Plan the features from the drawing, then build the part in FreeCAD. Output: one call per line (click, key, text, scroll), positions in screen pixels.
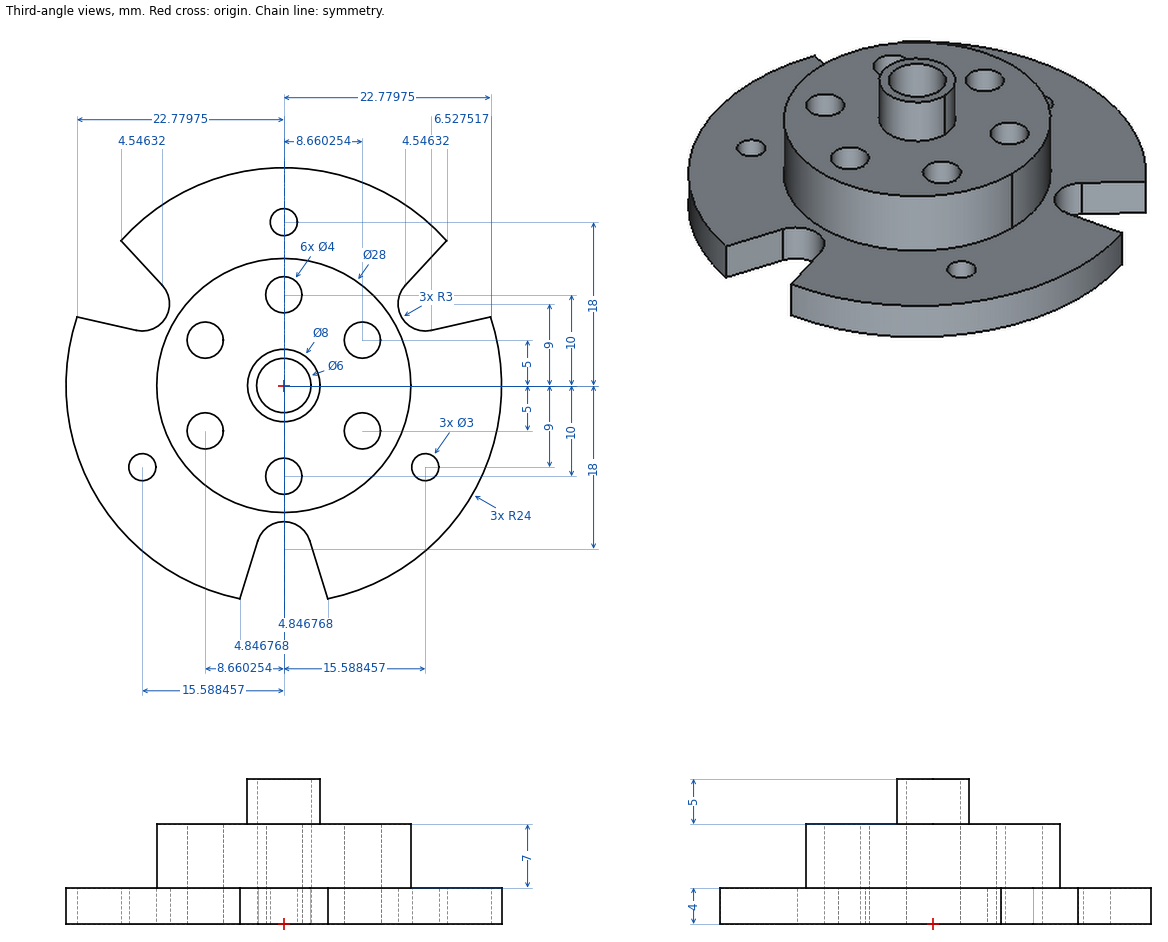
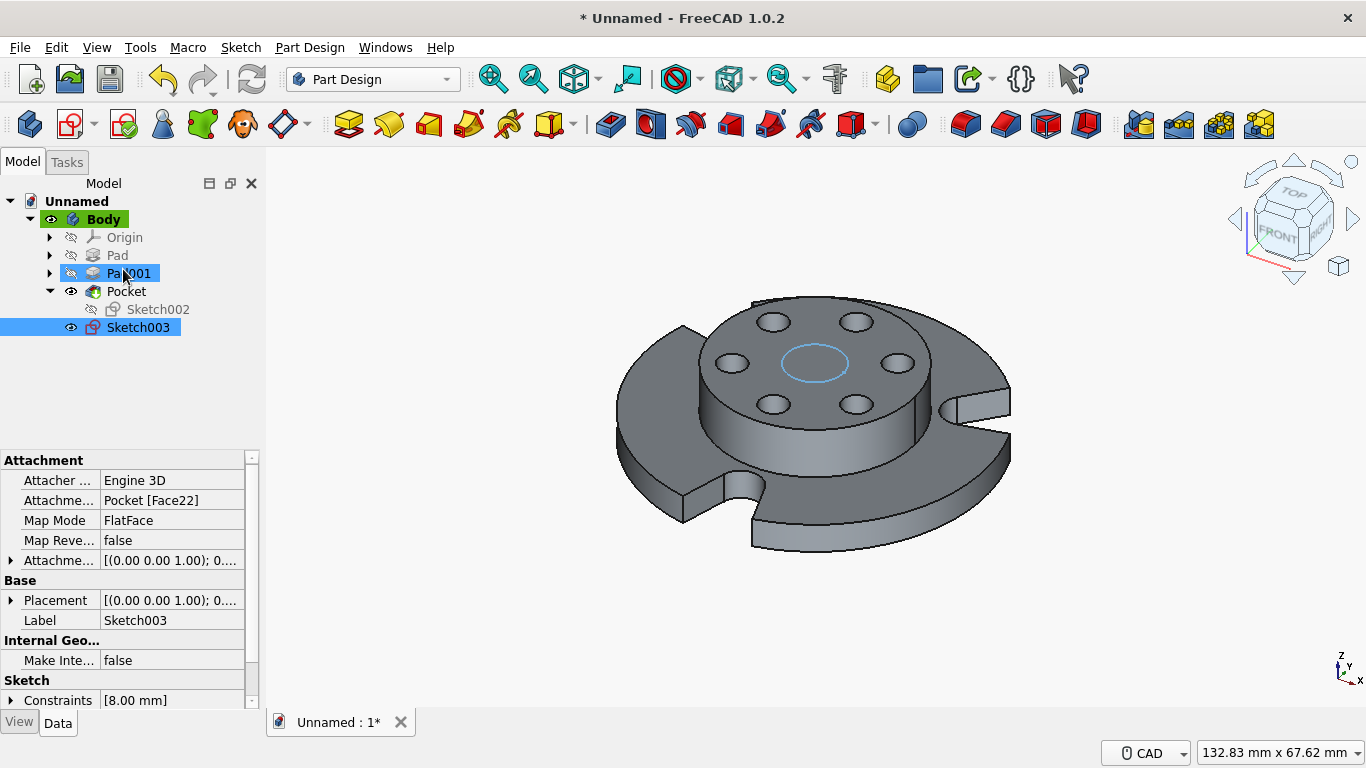
click(350, 124)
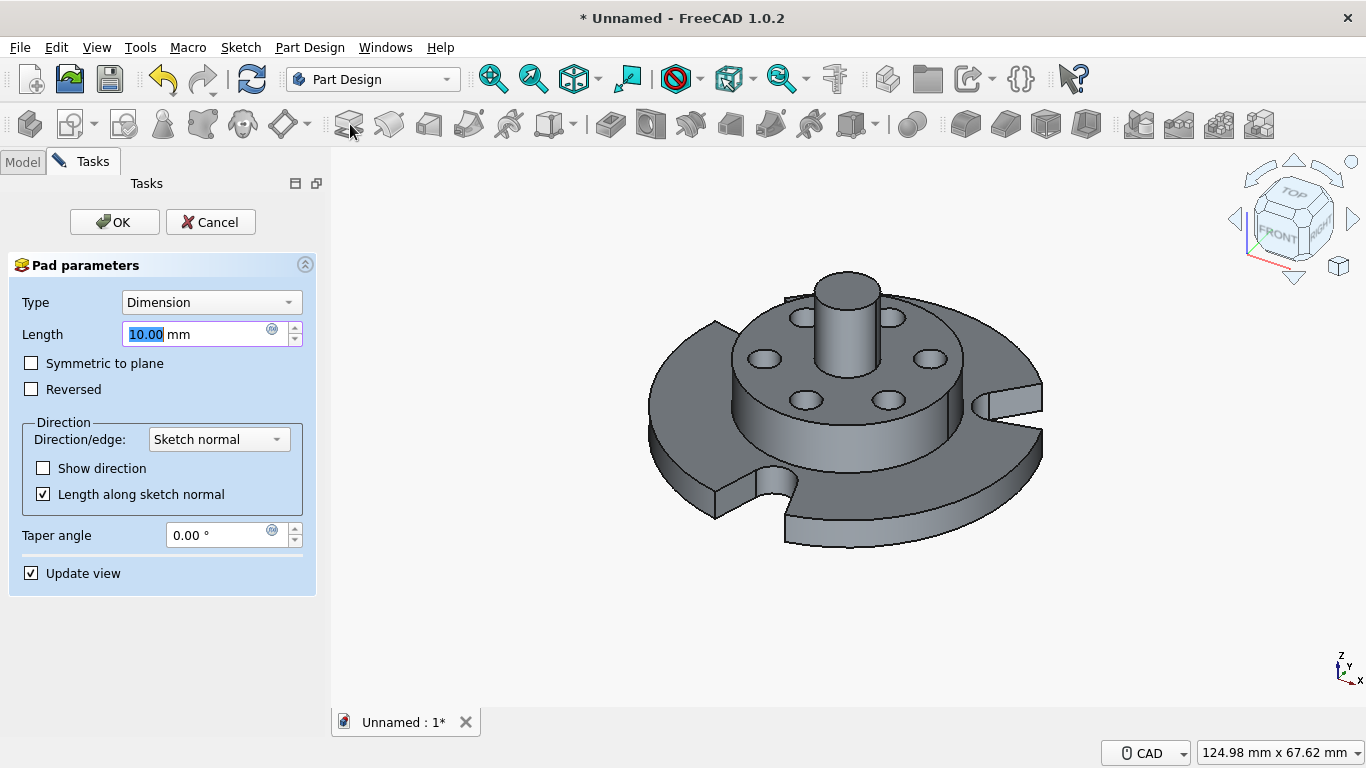
text(5)
key(Tab)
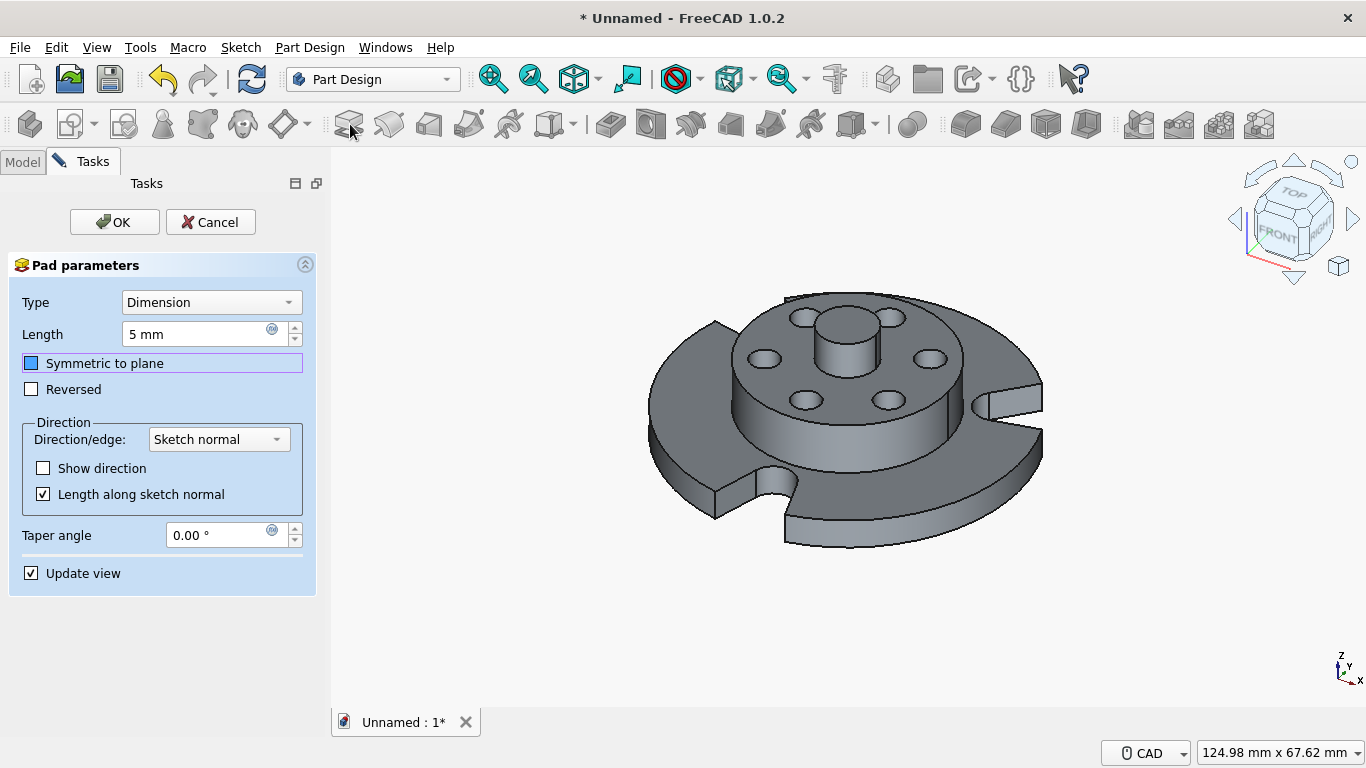
click(115, 222)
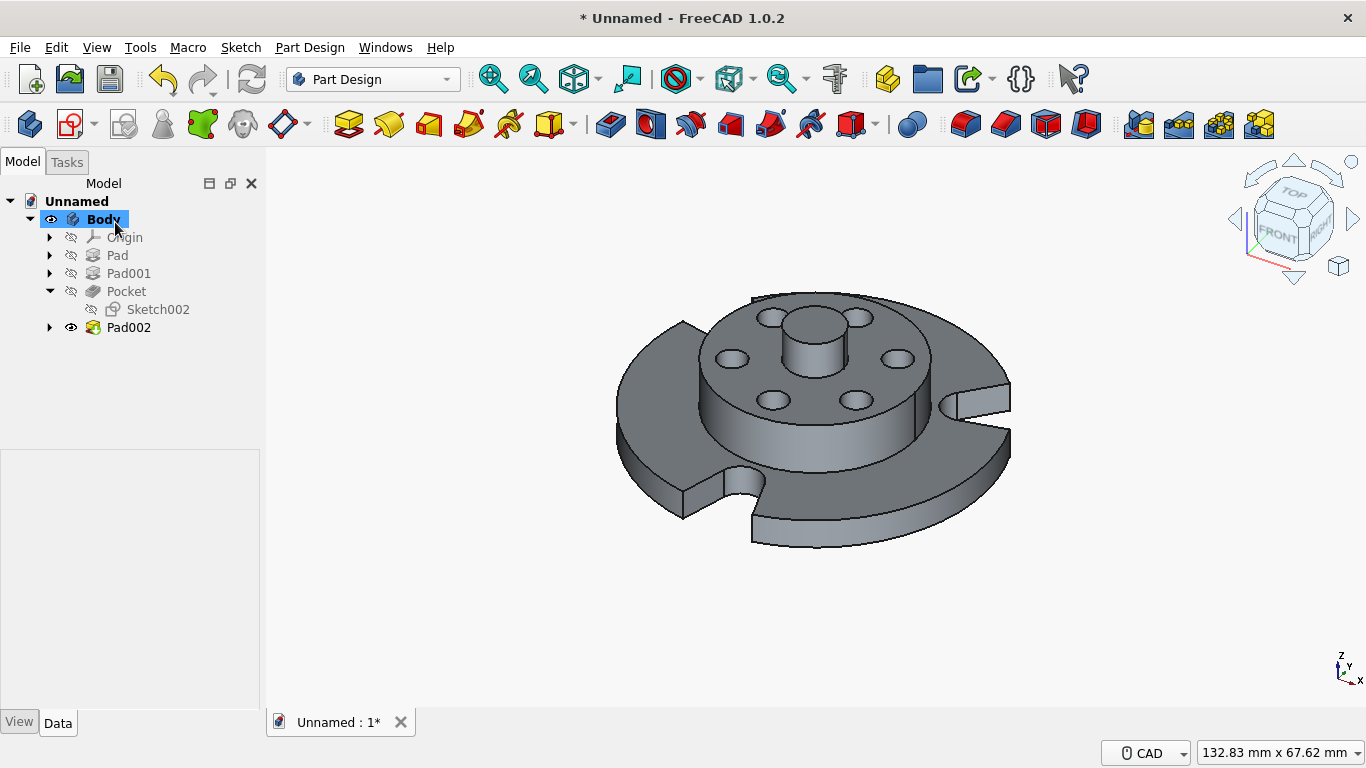
click(815, 324)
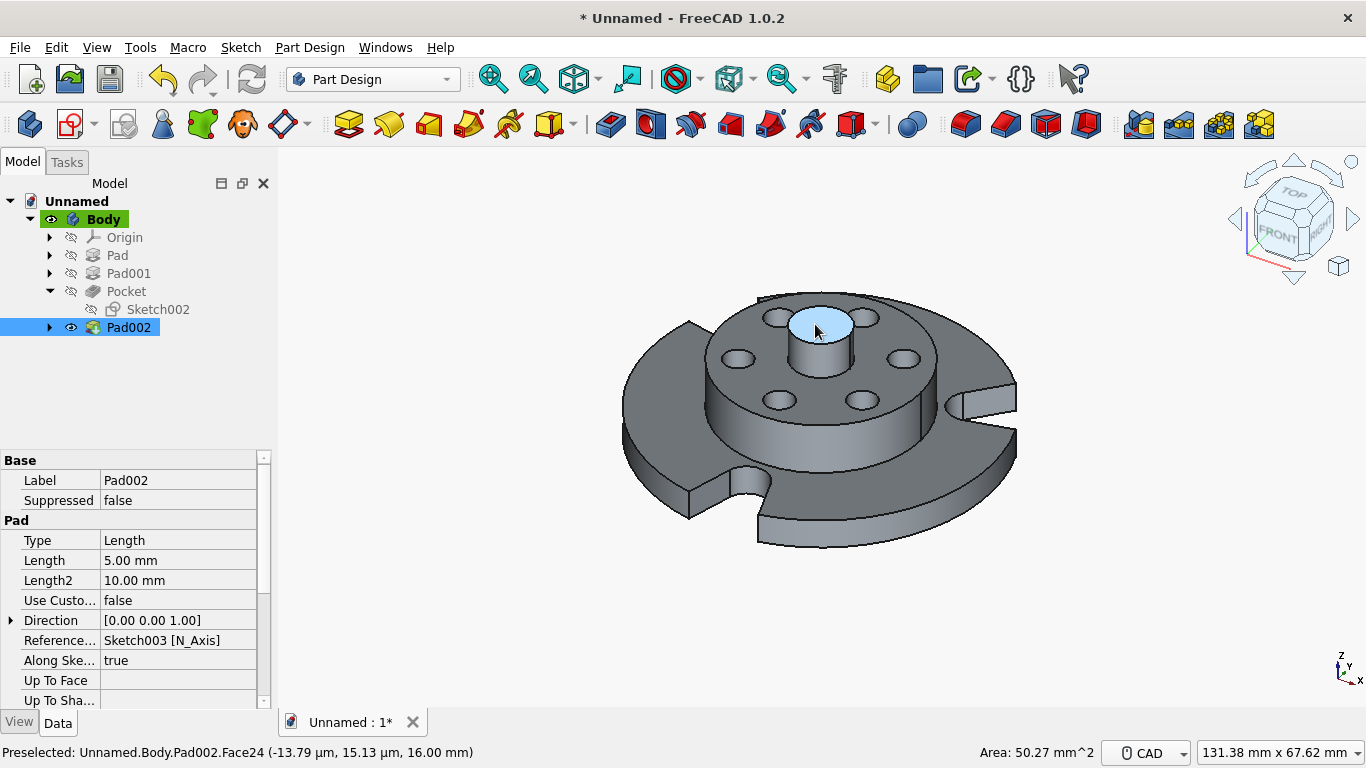
click(70, 124)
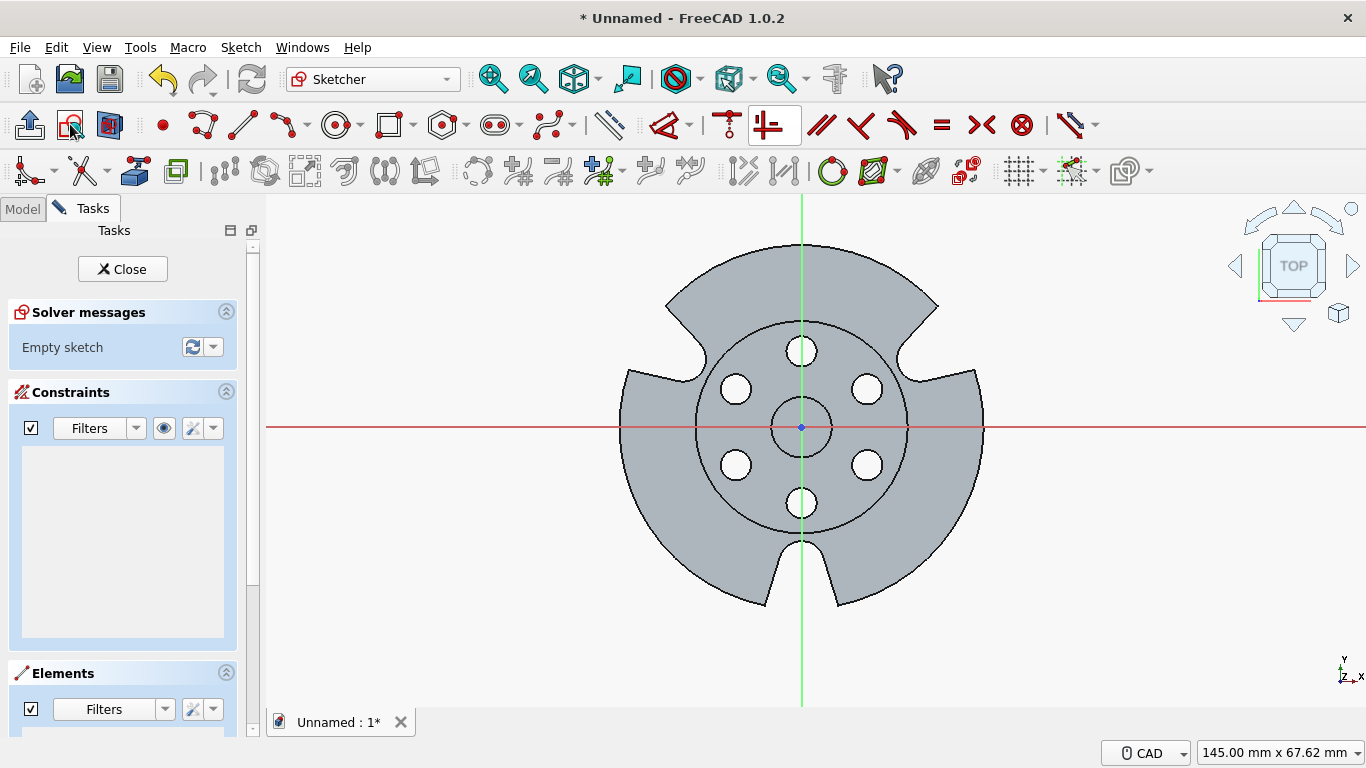
scroll(810, 424, up, 10)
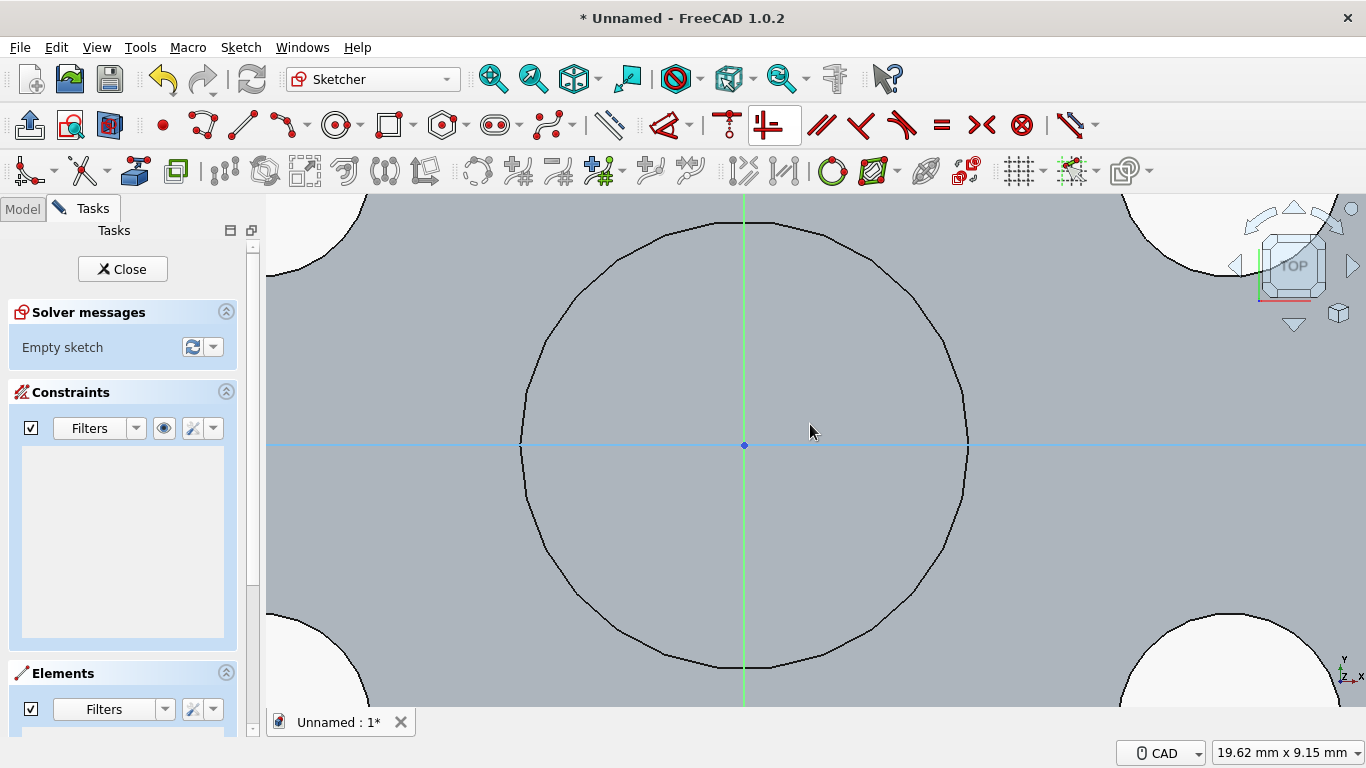
key(g)
key(c)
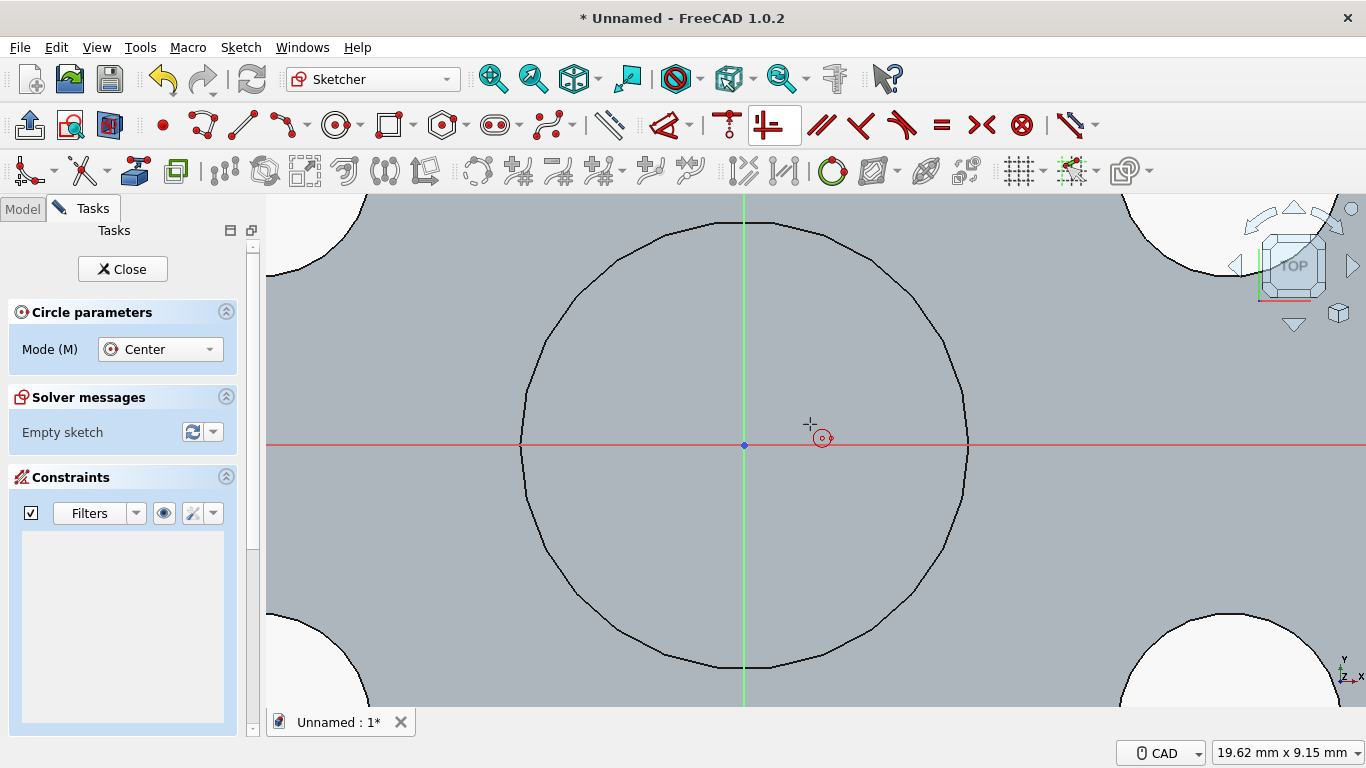
click(744, 445)
click(863, 326)
key(Escape)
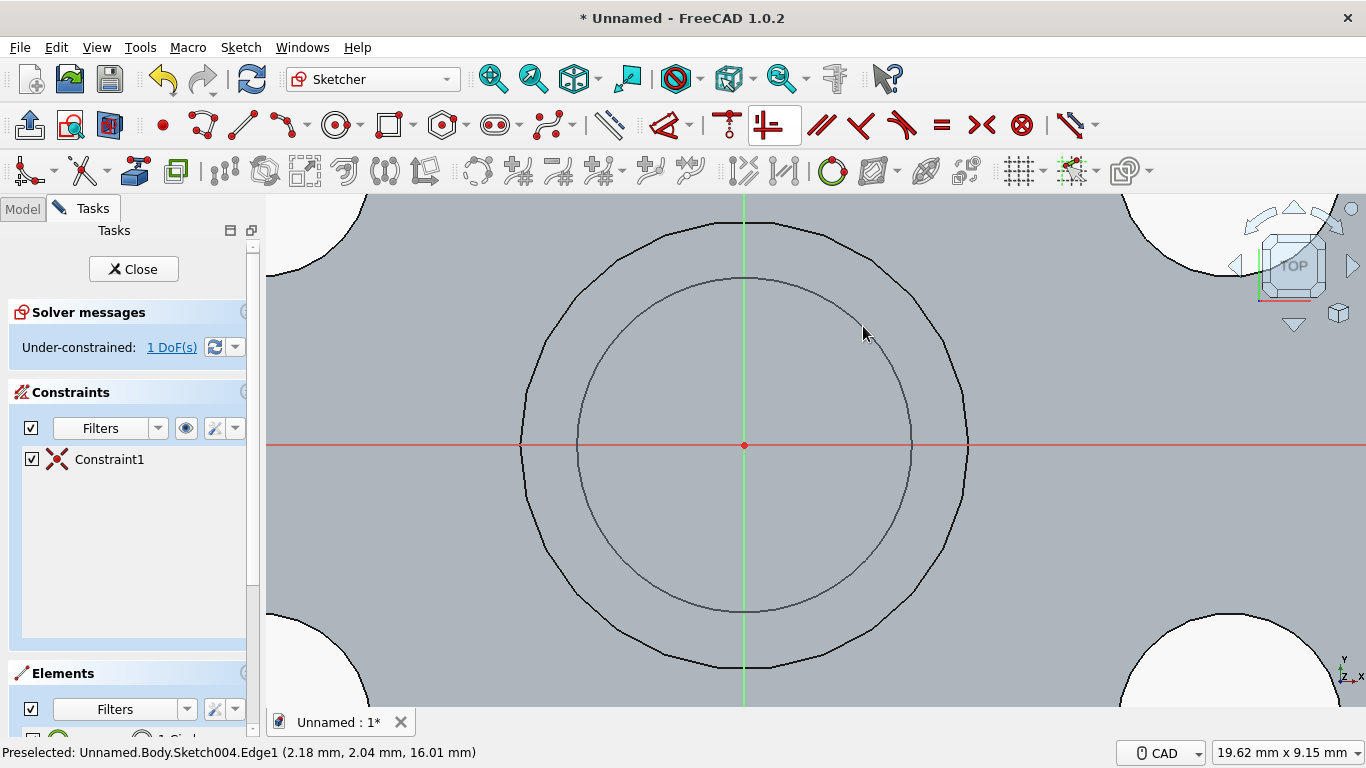
click(664, 126)